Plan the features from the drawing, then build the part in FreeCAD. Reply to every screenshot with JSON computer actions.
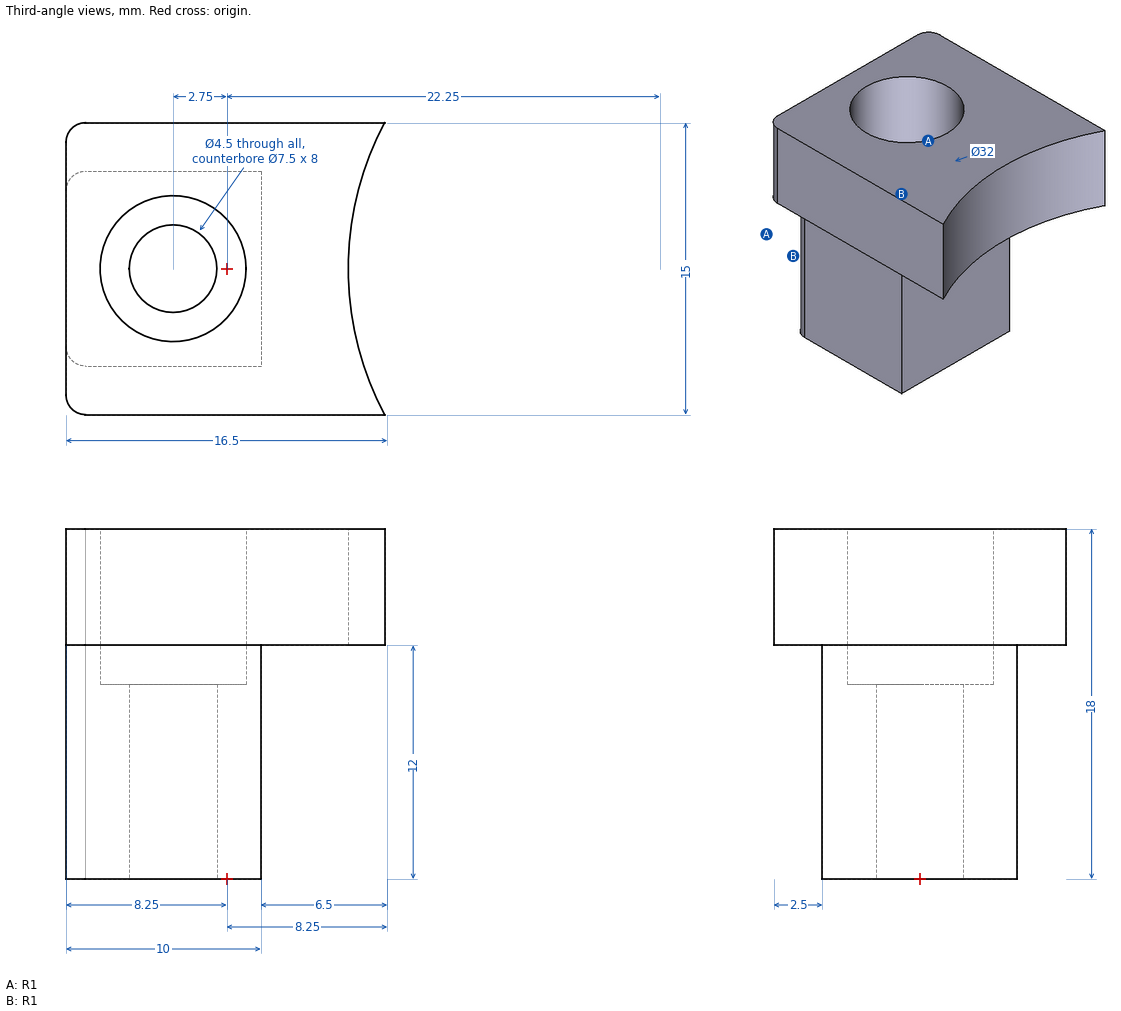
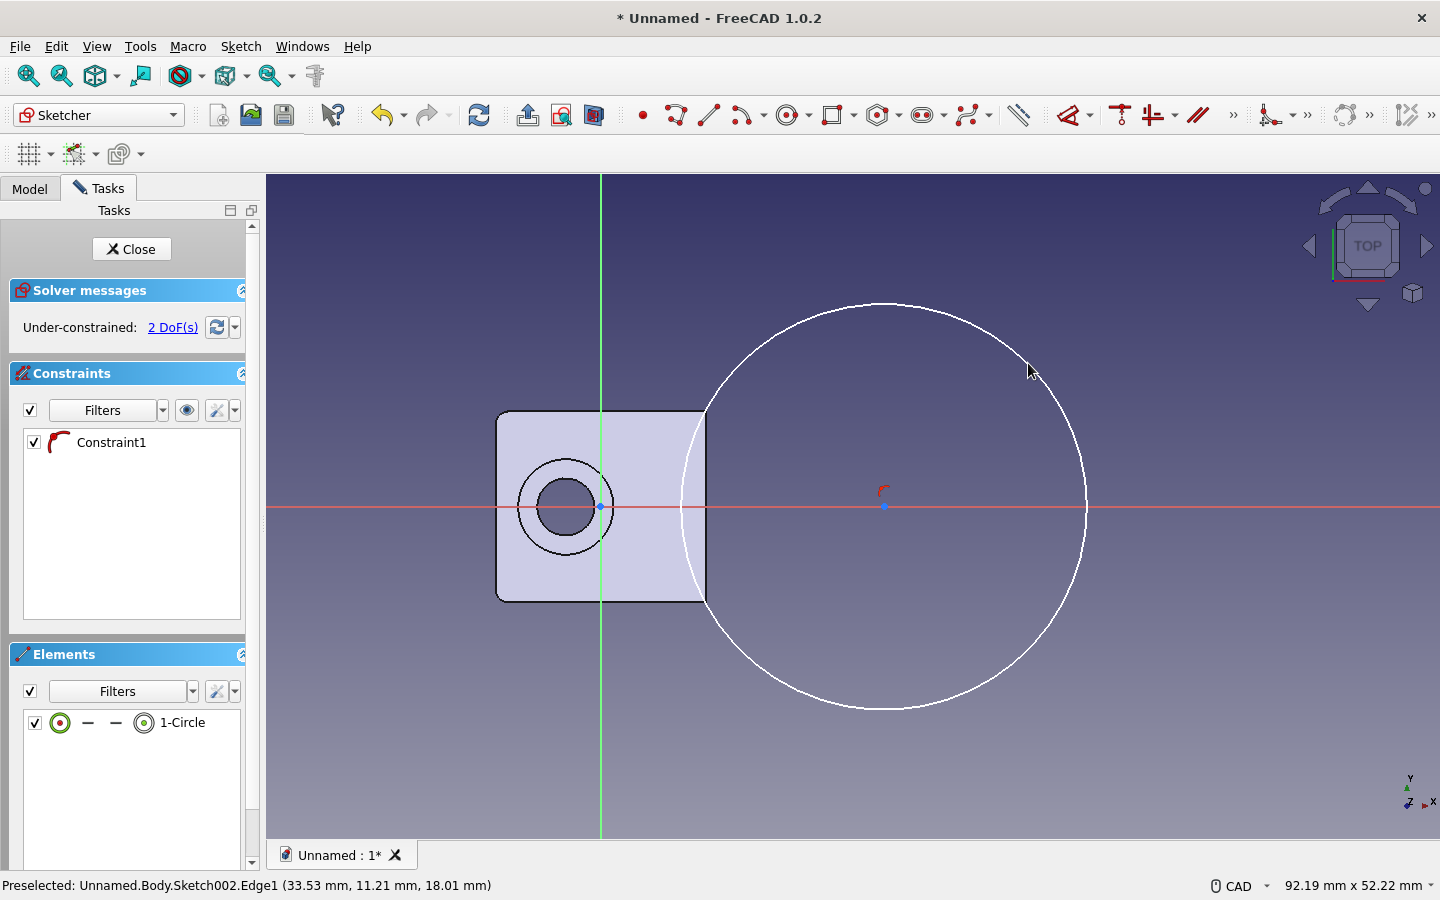
{"action": "key", "text": "d"}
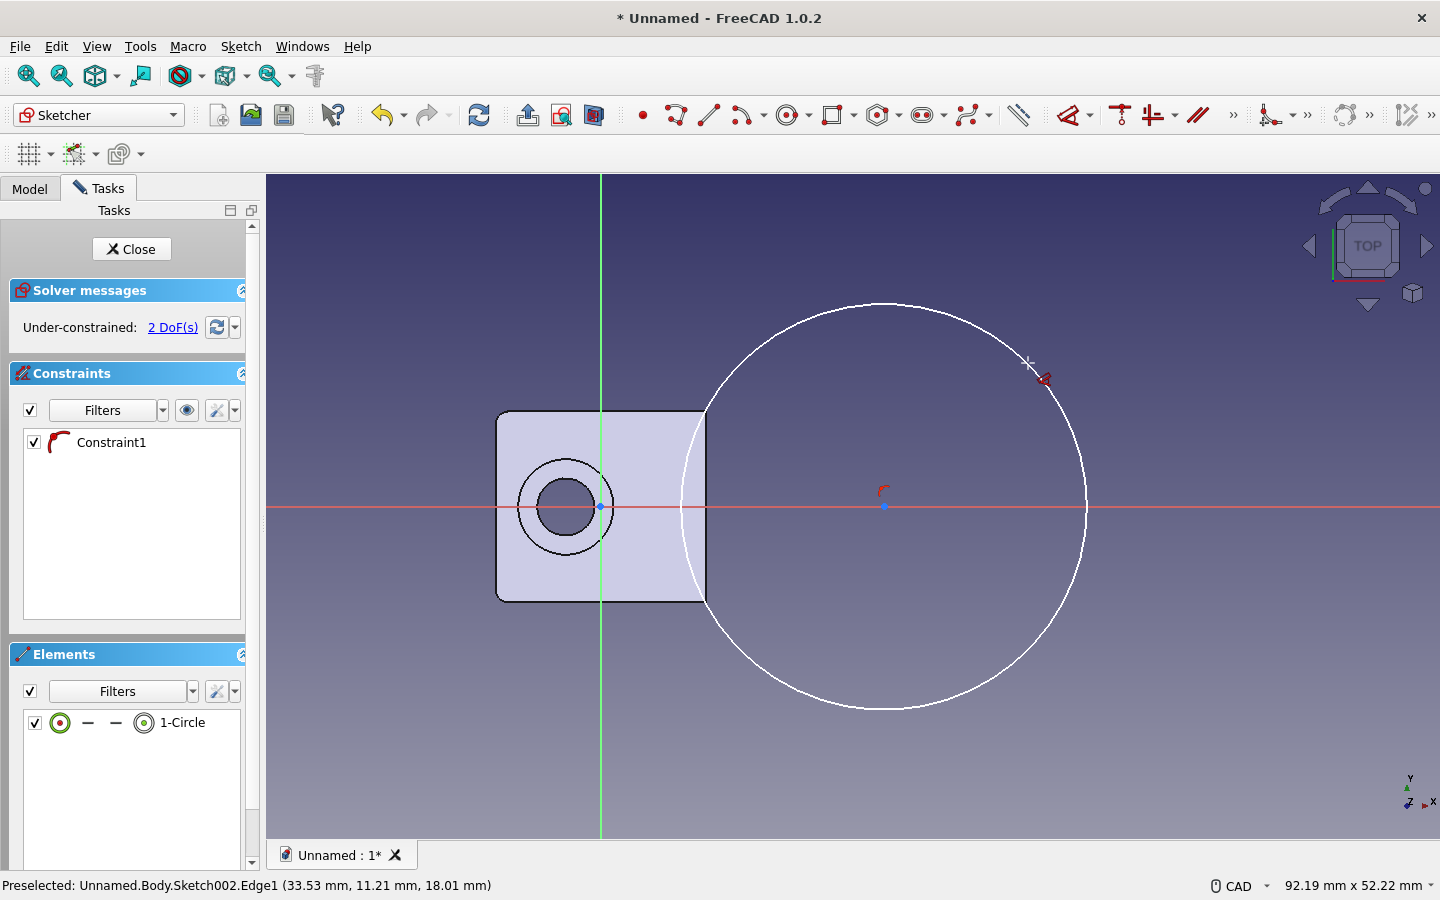
{"action": "left_click", "coordinate": [1027, 363]}
{"action": "left_click", "coordinate": [1050, 340]}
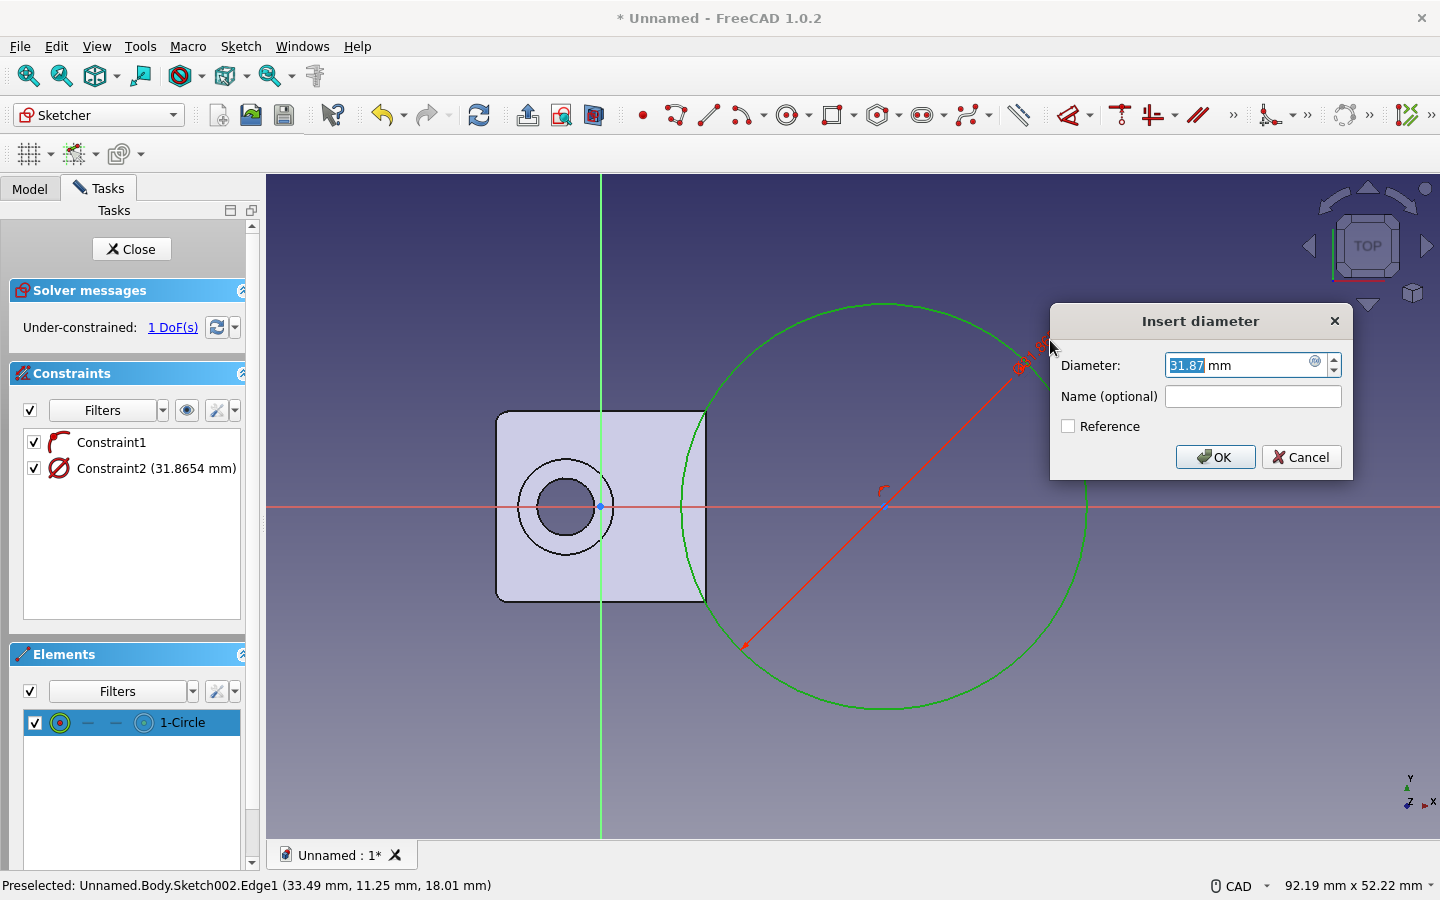
{"action": "type", "text": "32"}
{"action": "key", "text": "Return"}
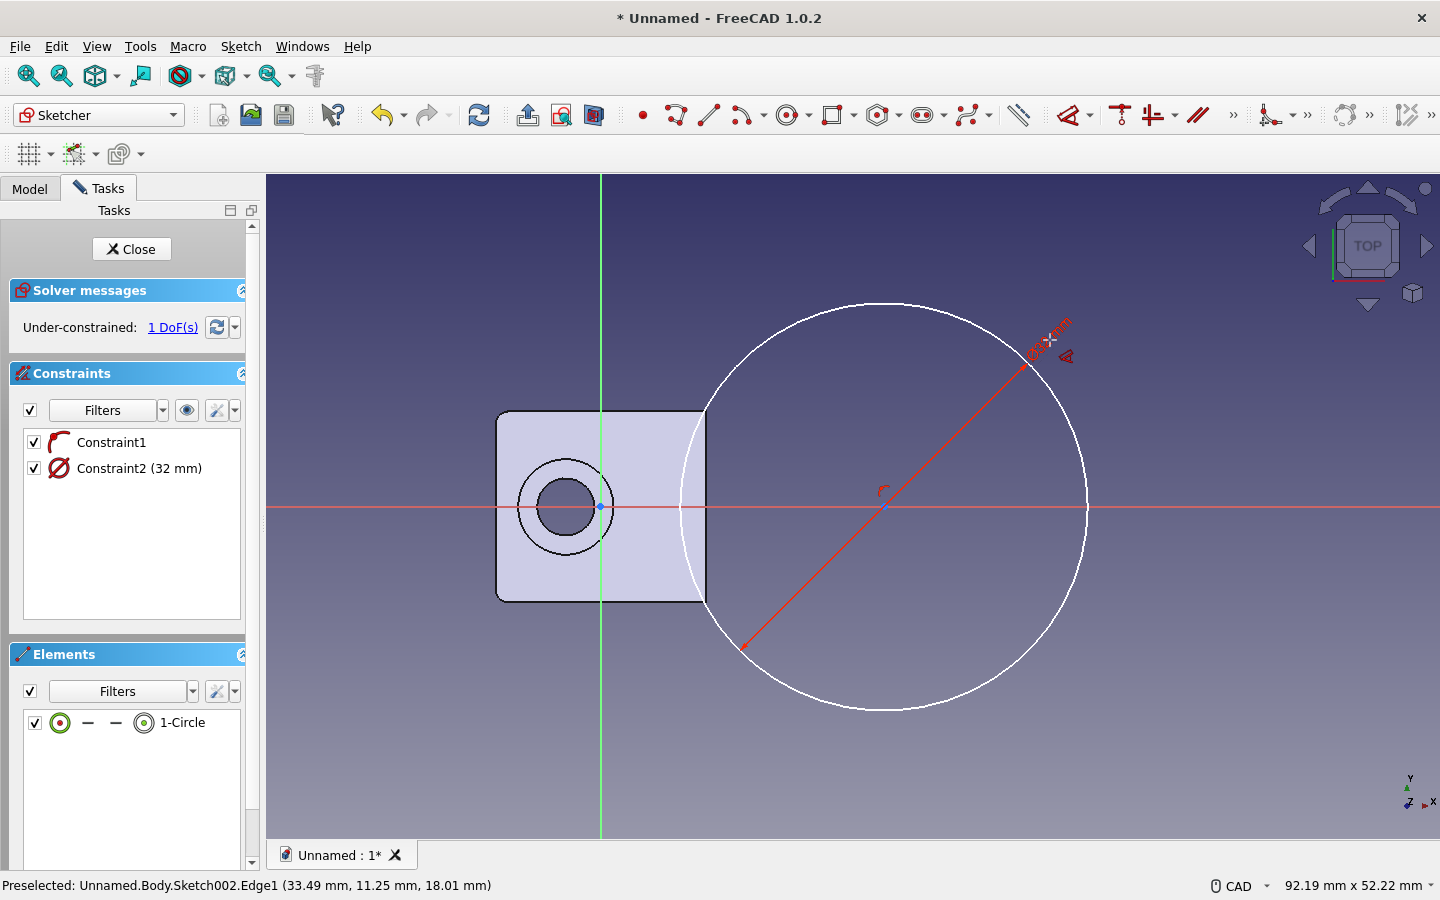
{"action": "left_click", "coordinate": [884, 507]}
{"action": "left_click", "coordinate": [742, 541]}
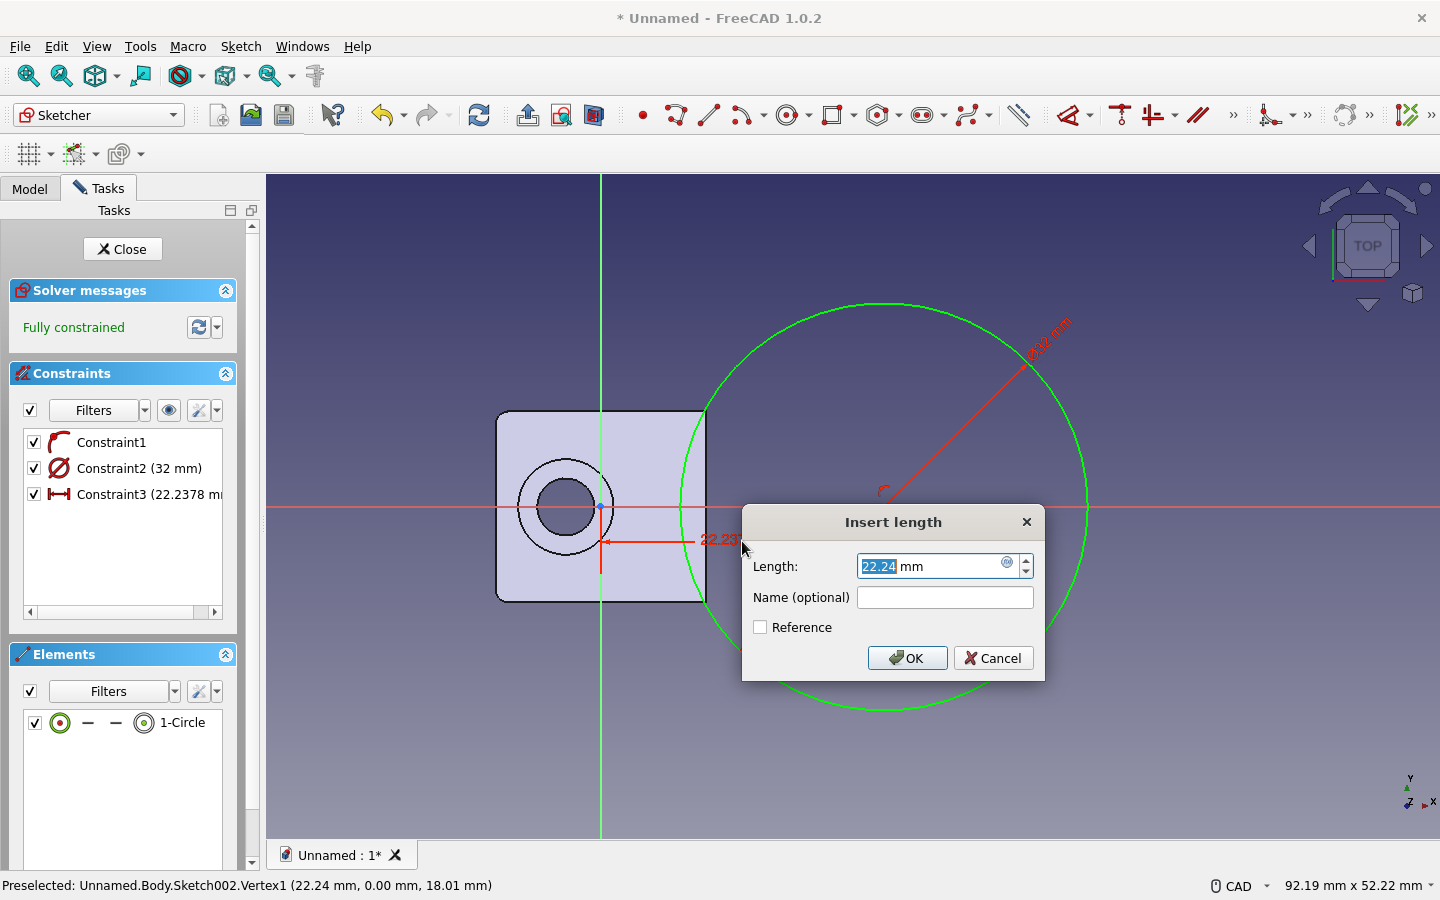
{"action": "type", "text": "22.25"}
{"action": "key", "text": "Return"}
{"action": "key", "text": "Escape"}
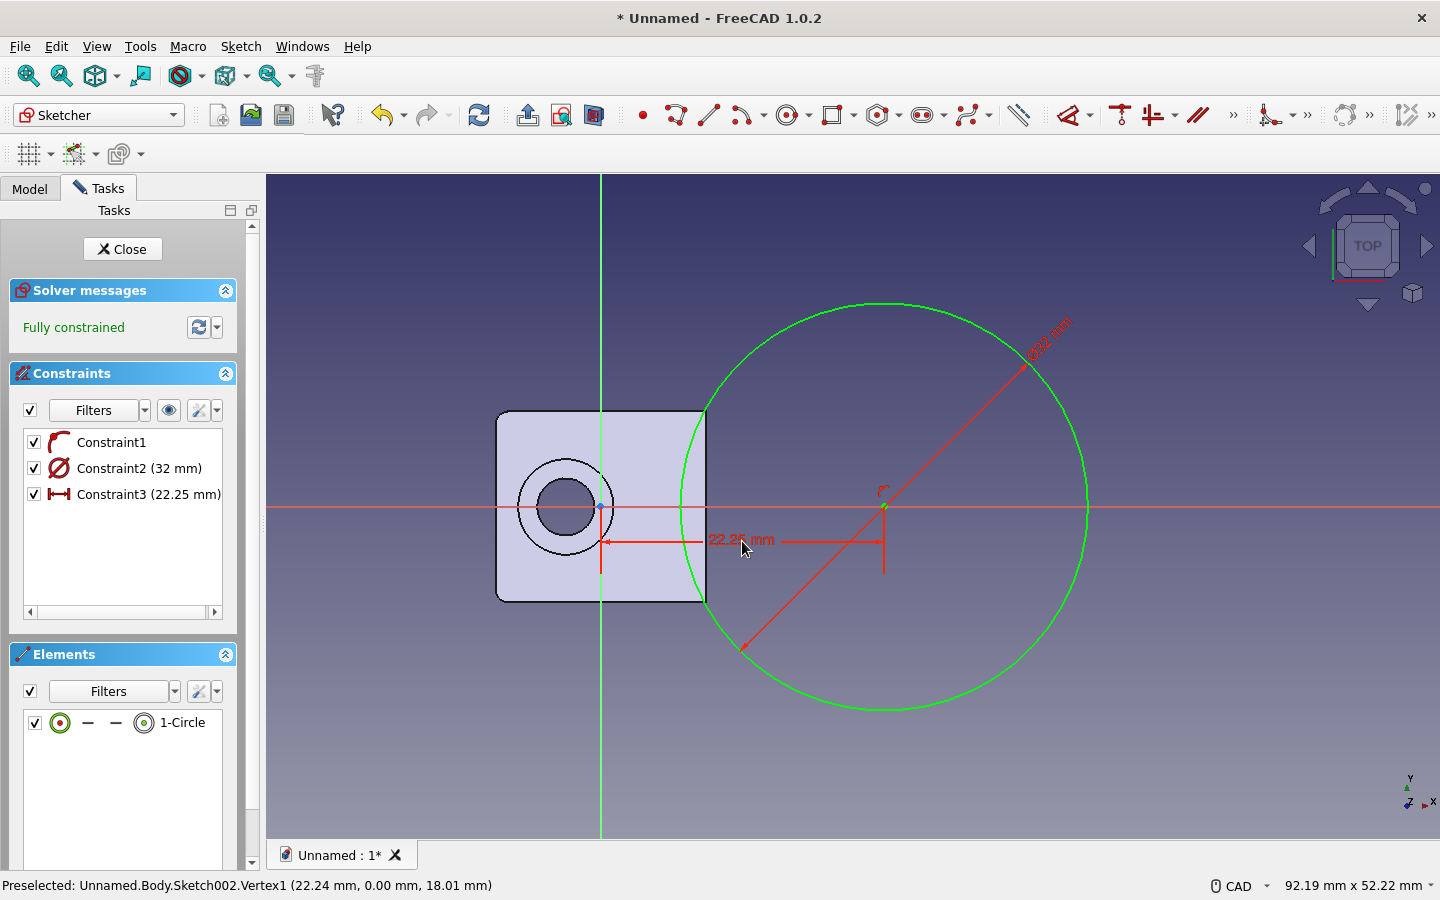
{"action": "left_click", "coordinate": [123, 249]}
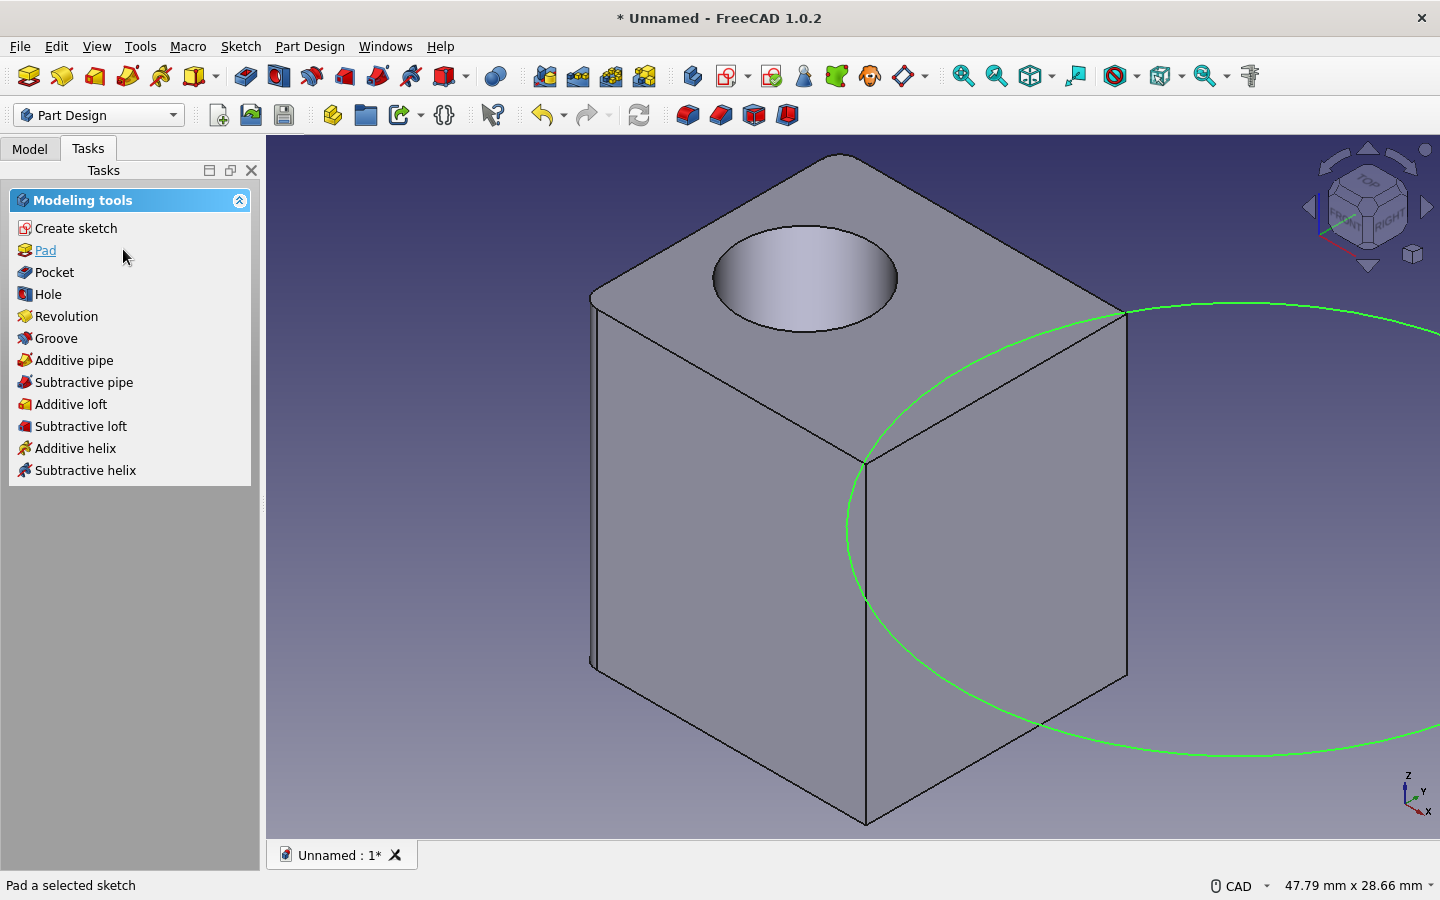
{"action": "left_click", "coordinate": [246, 76]}